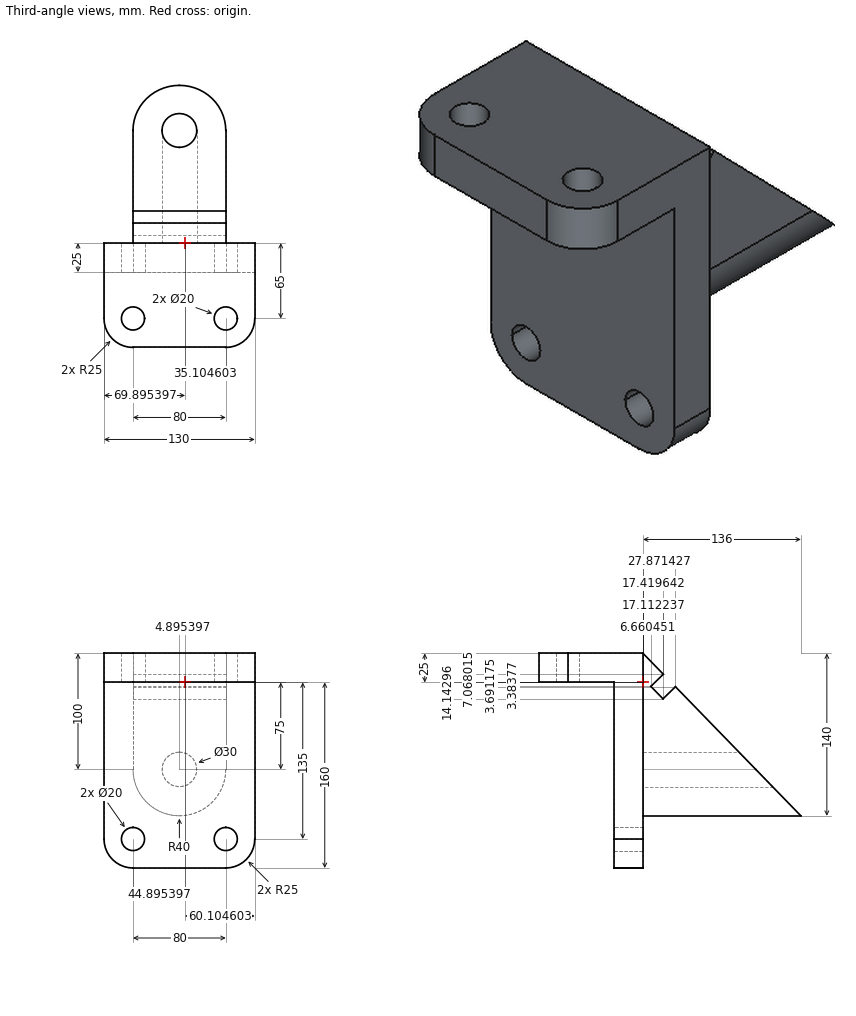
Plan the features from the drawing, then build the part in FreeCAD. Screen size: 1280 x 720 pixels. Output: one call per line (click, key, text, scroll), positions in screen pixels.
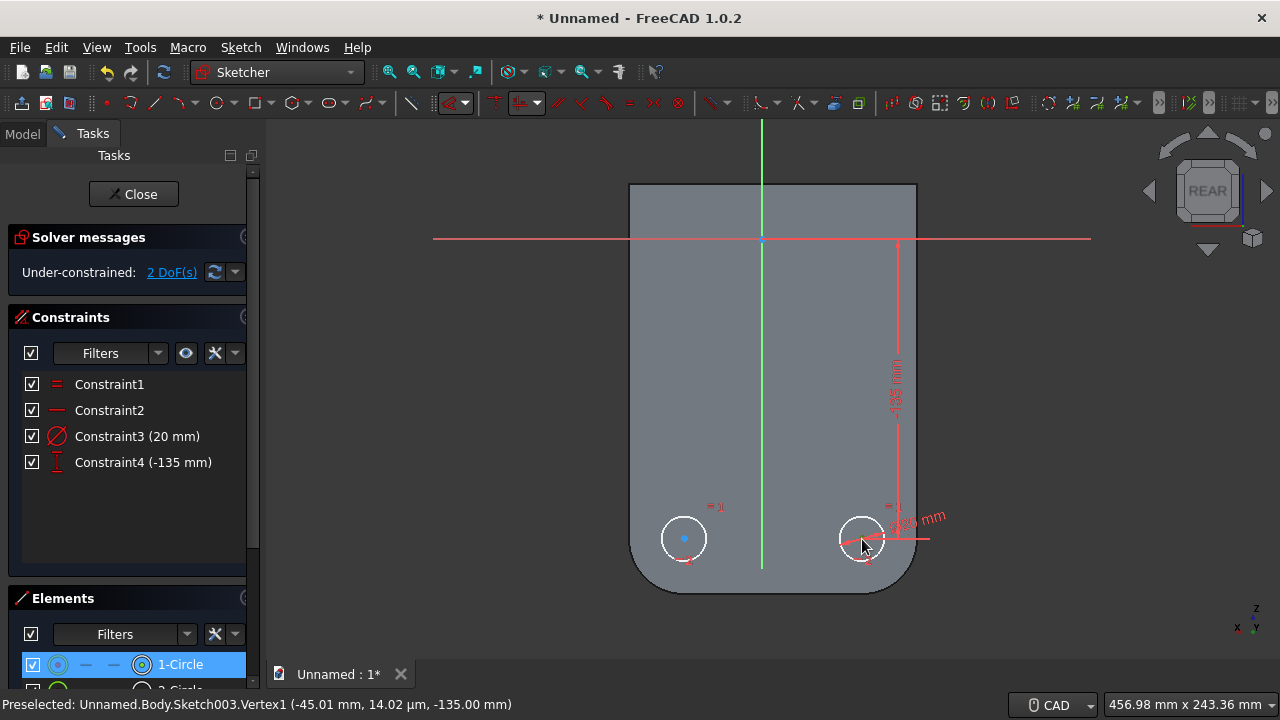
click(684, 539)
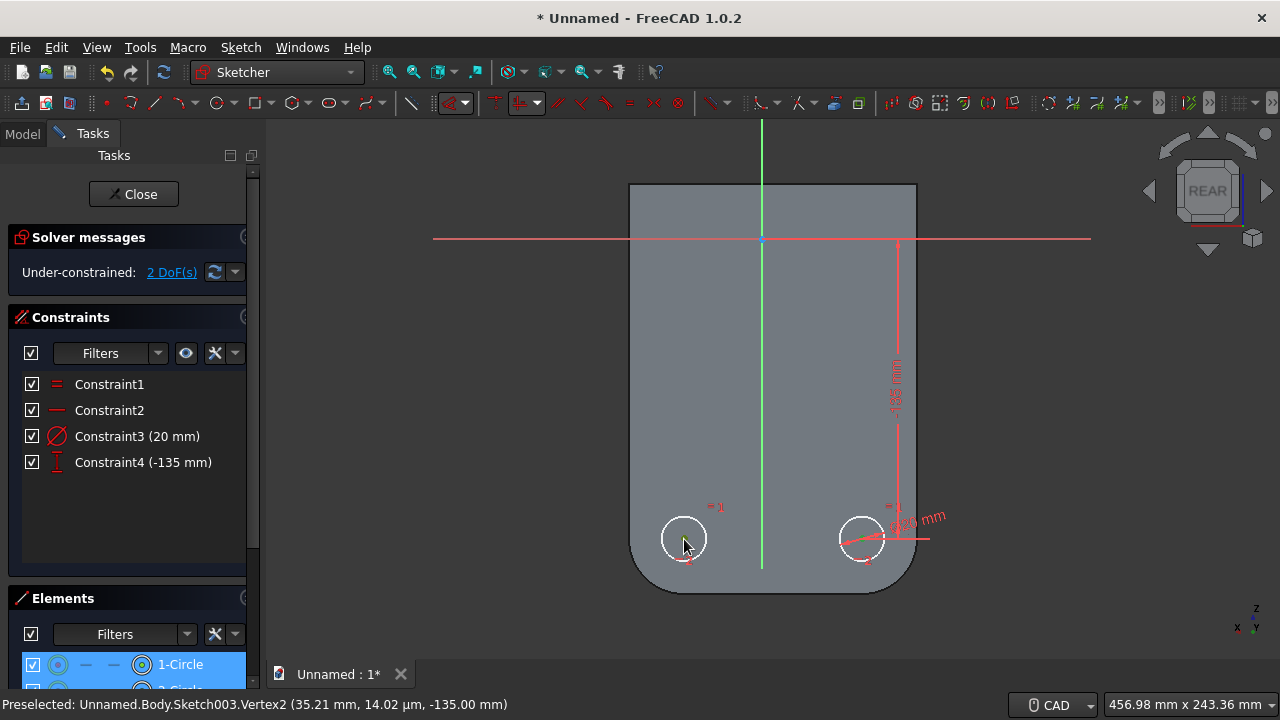
click(468, 104)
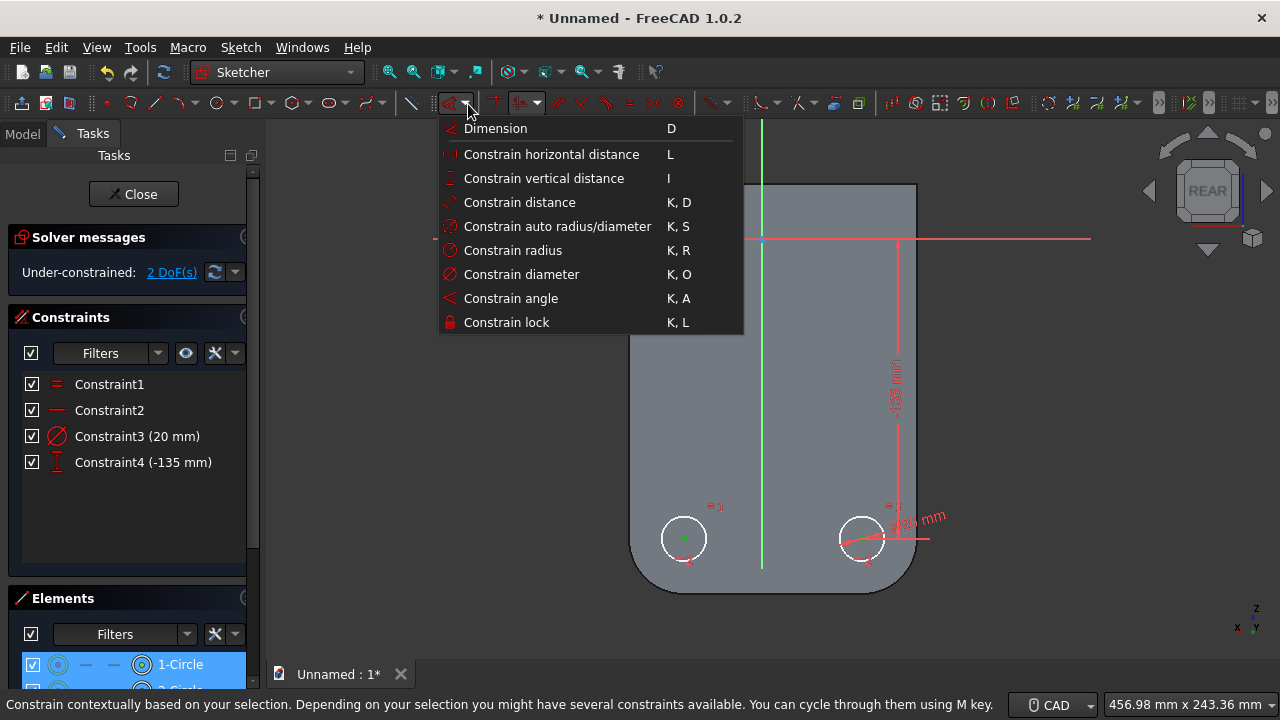
click(591, 154)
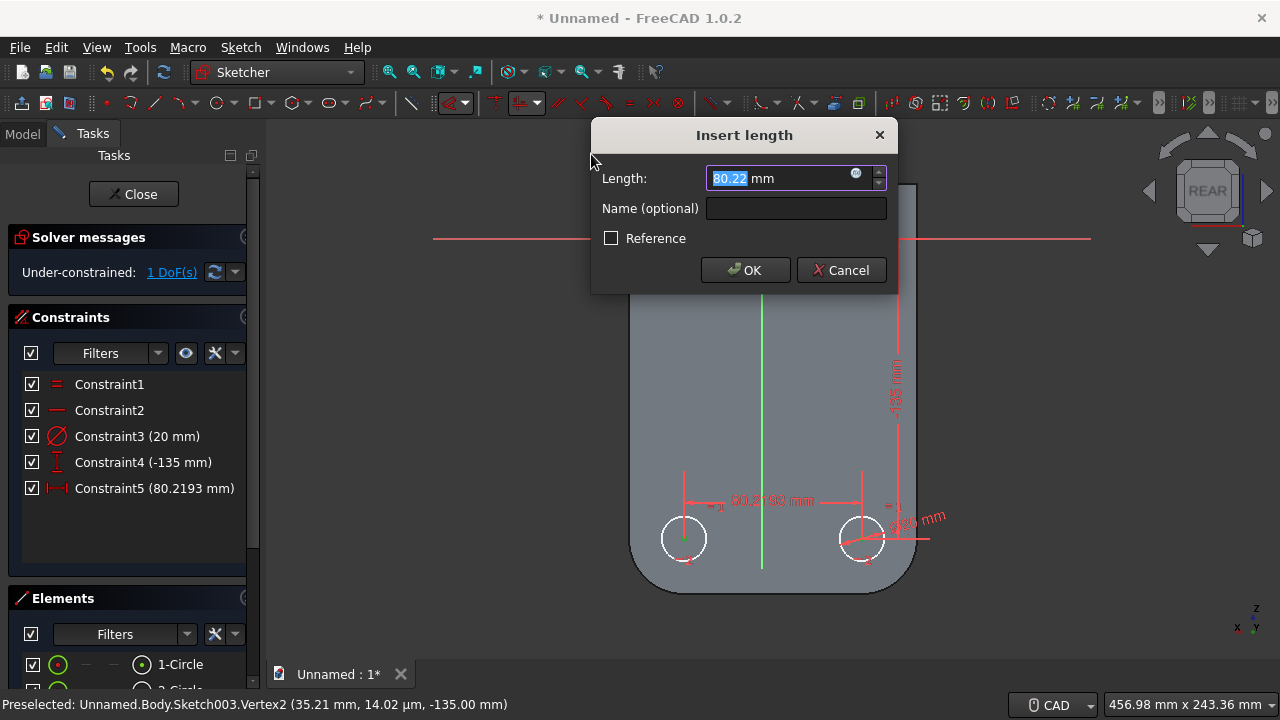
text(80)
key(Return)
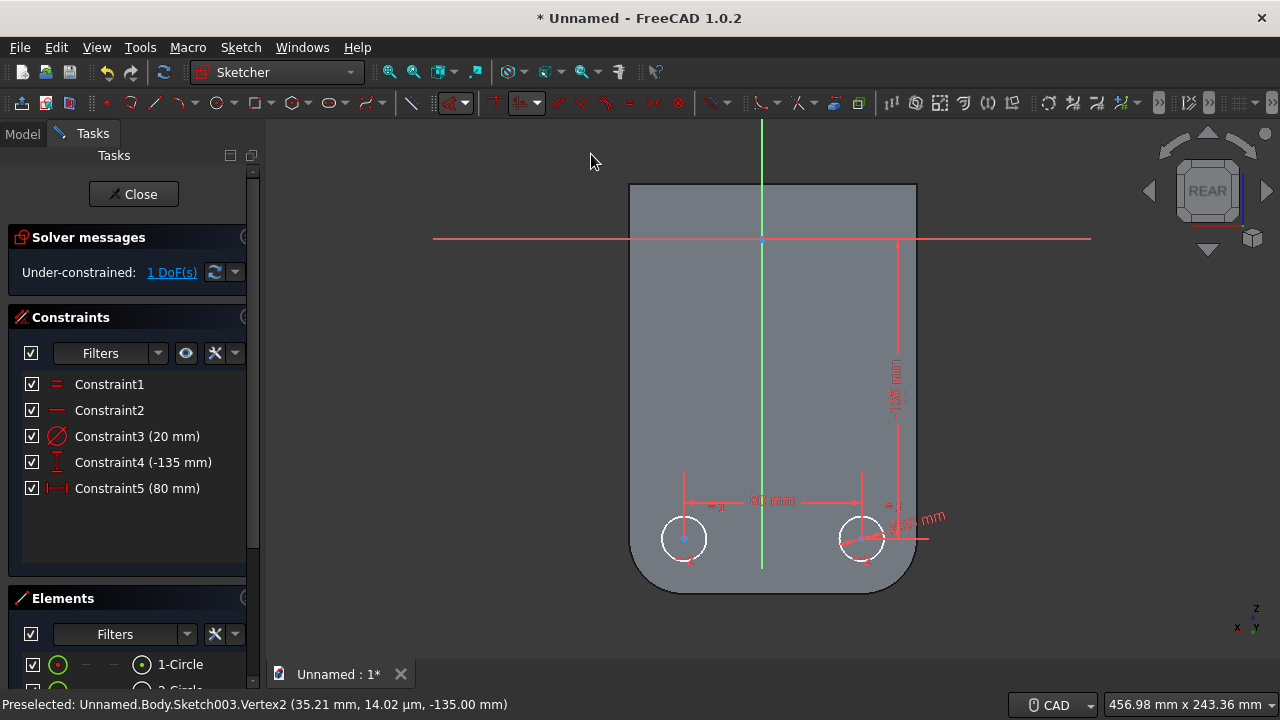
click(862, 539)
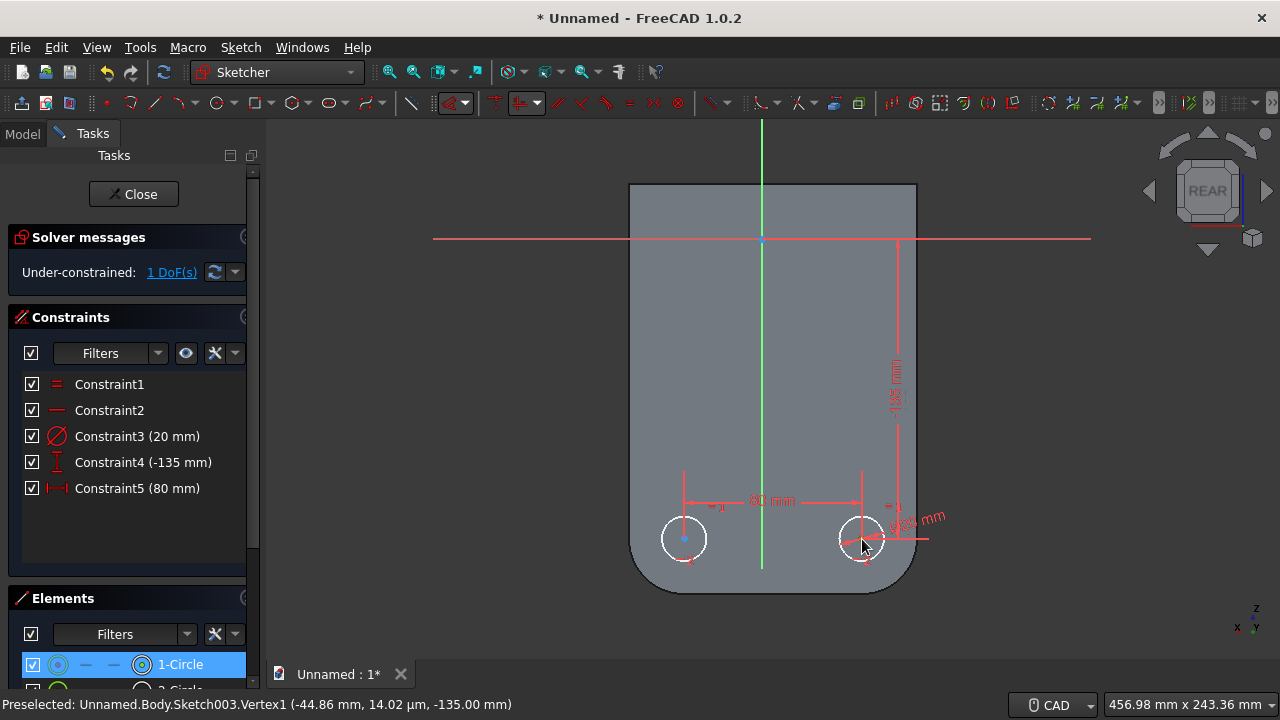
click(468, 104)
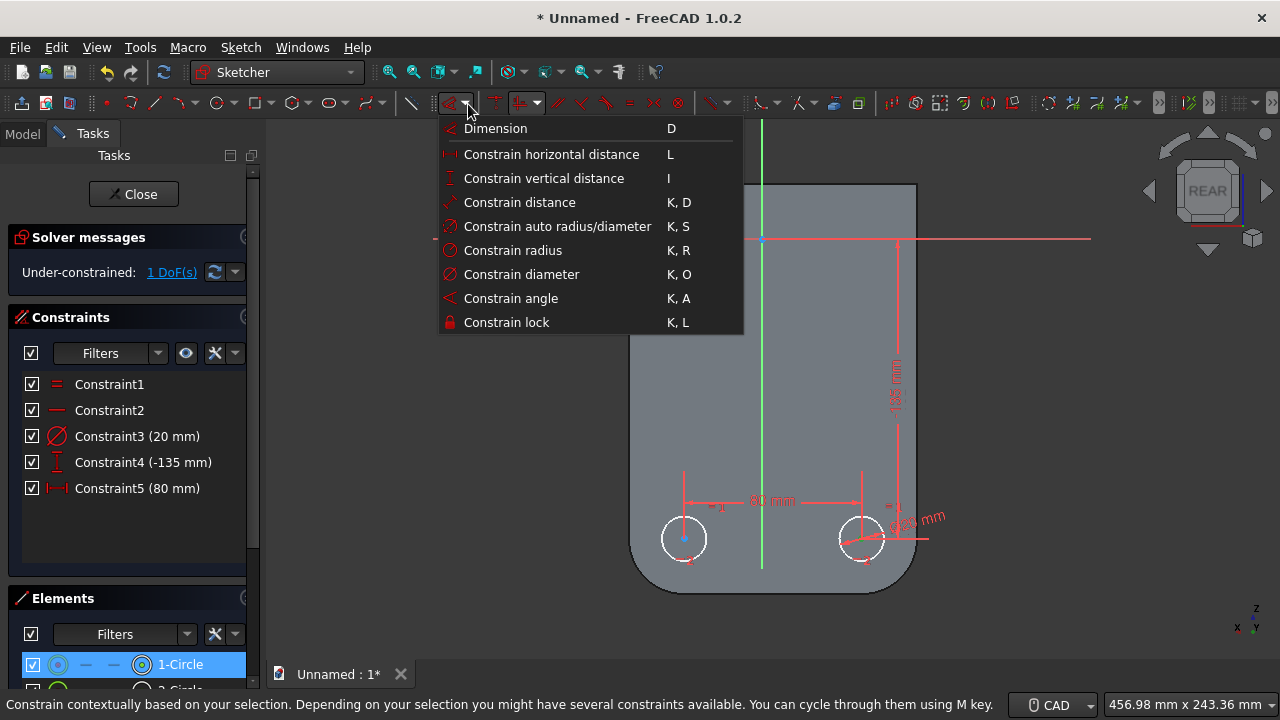
click(591, 154)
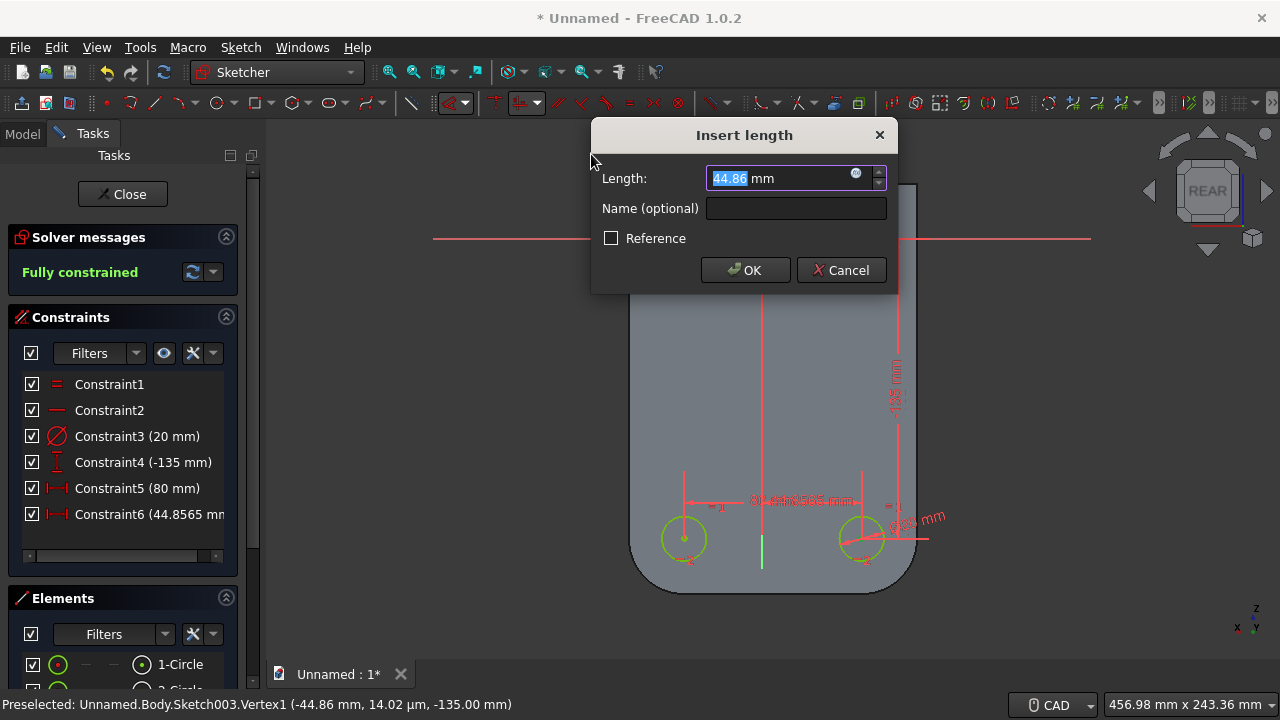
text(44.895397)
key(Return)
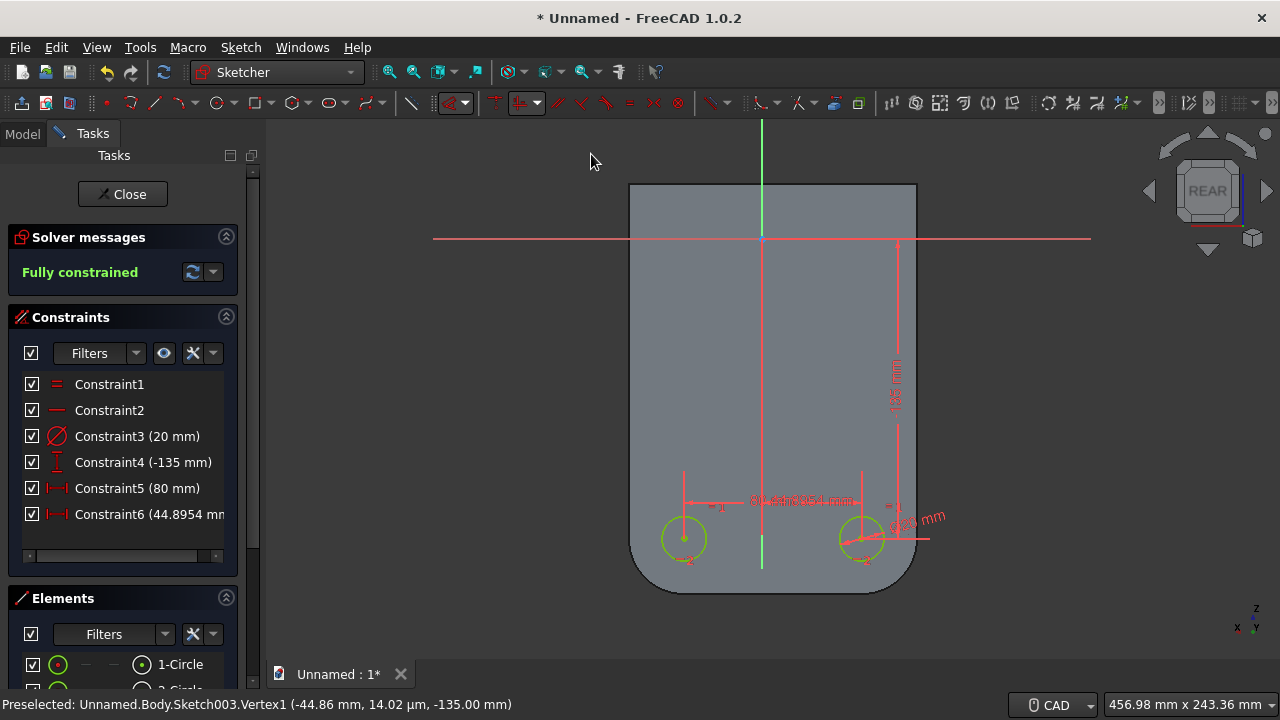
click(123, 194)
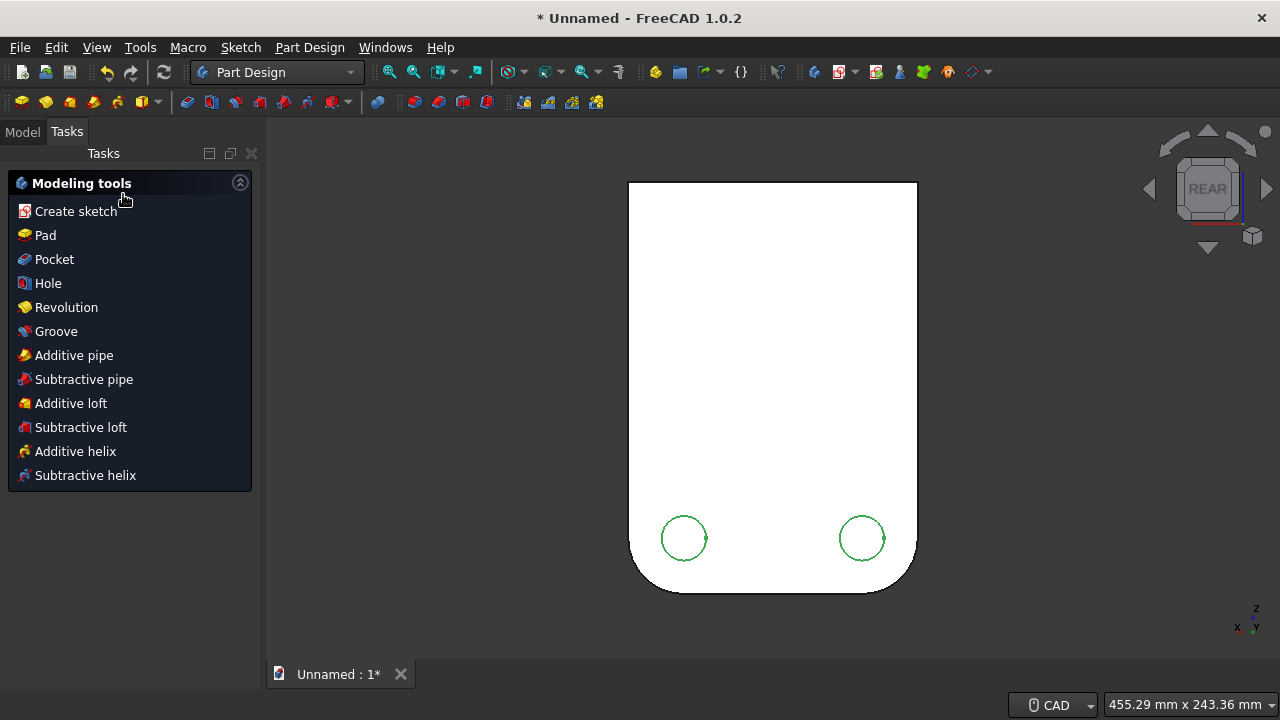
click(188, 102)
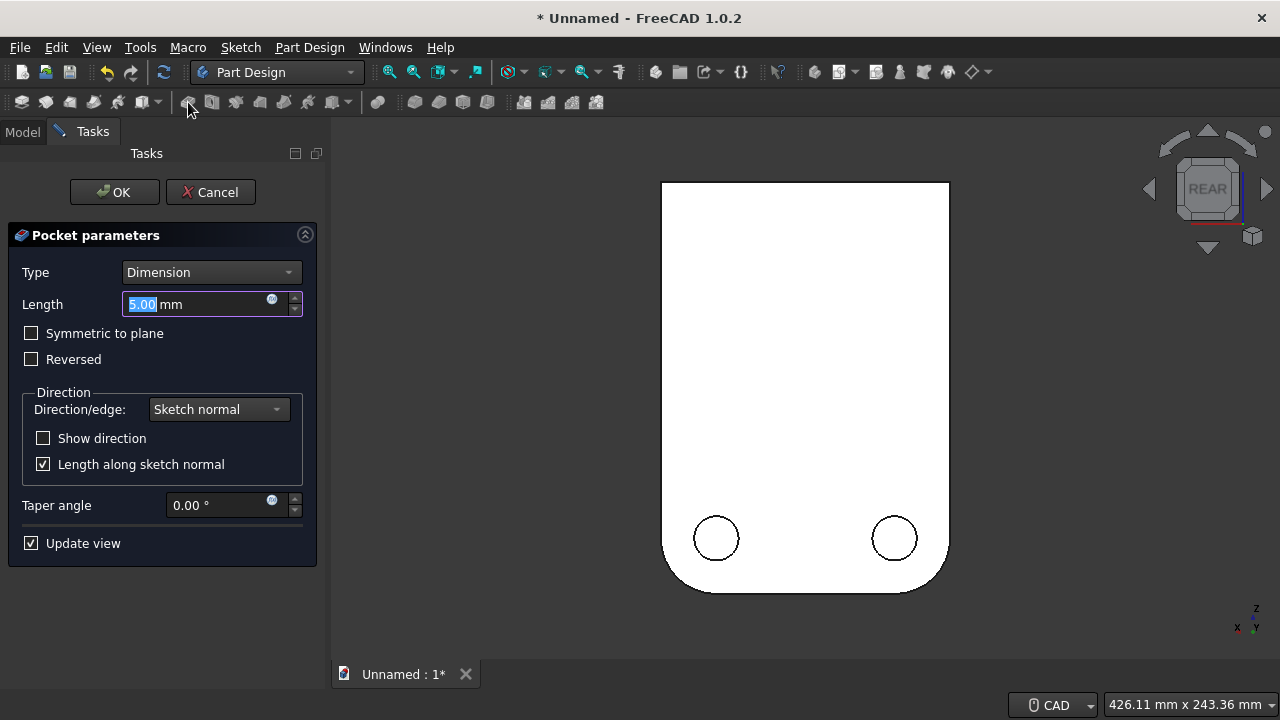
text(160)
key(Tab)